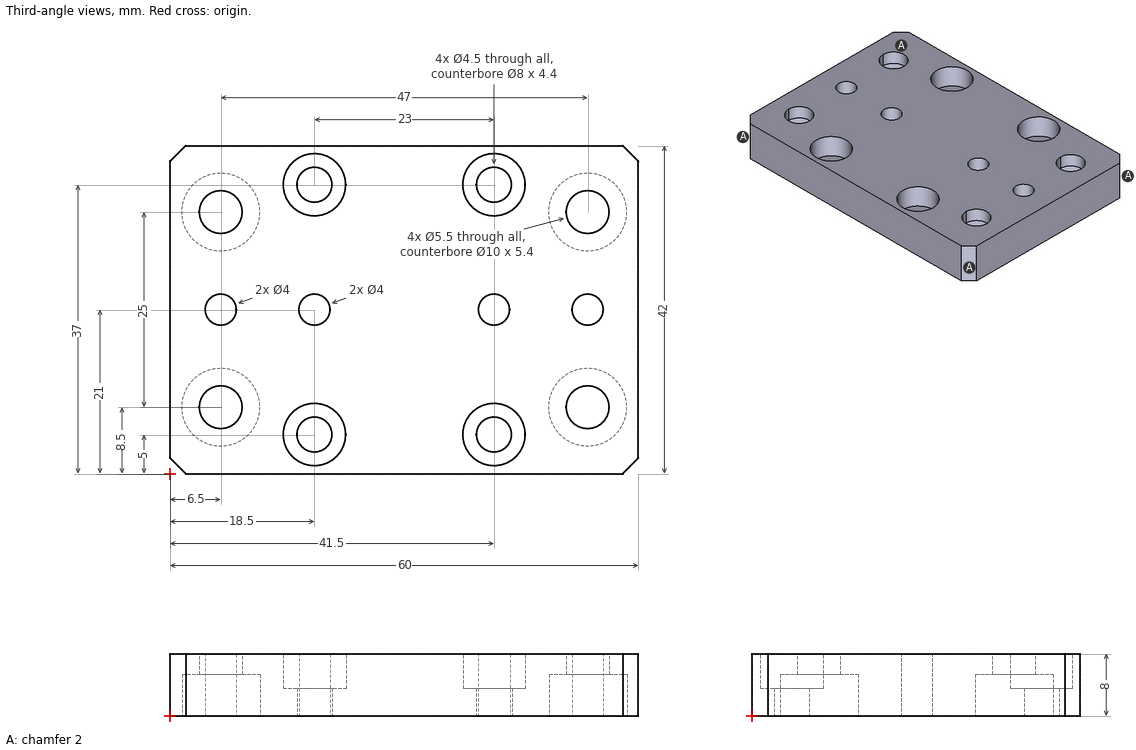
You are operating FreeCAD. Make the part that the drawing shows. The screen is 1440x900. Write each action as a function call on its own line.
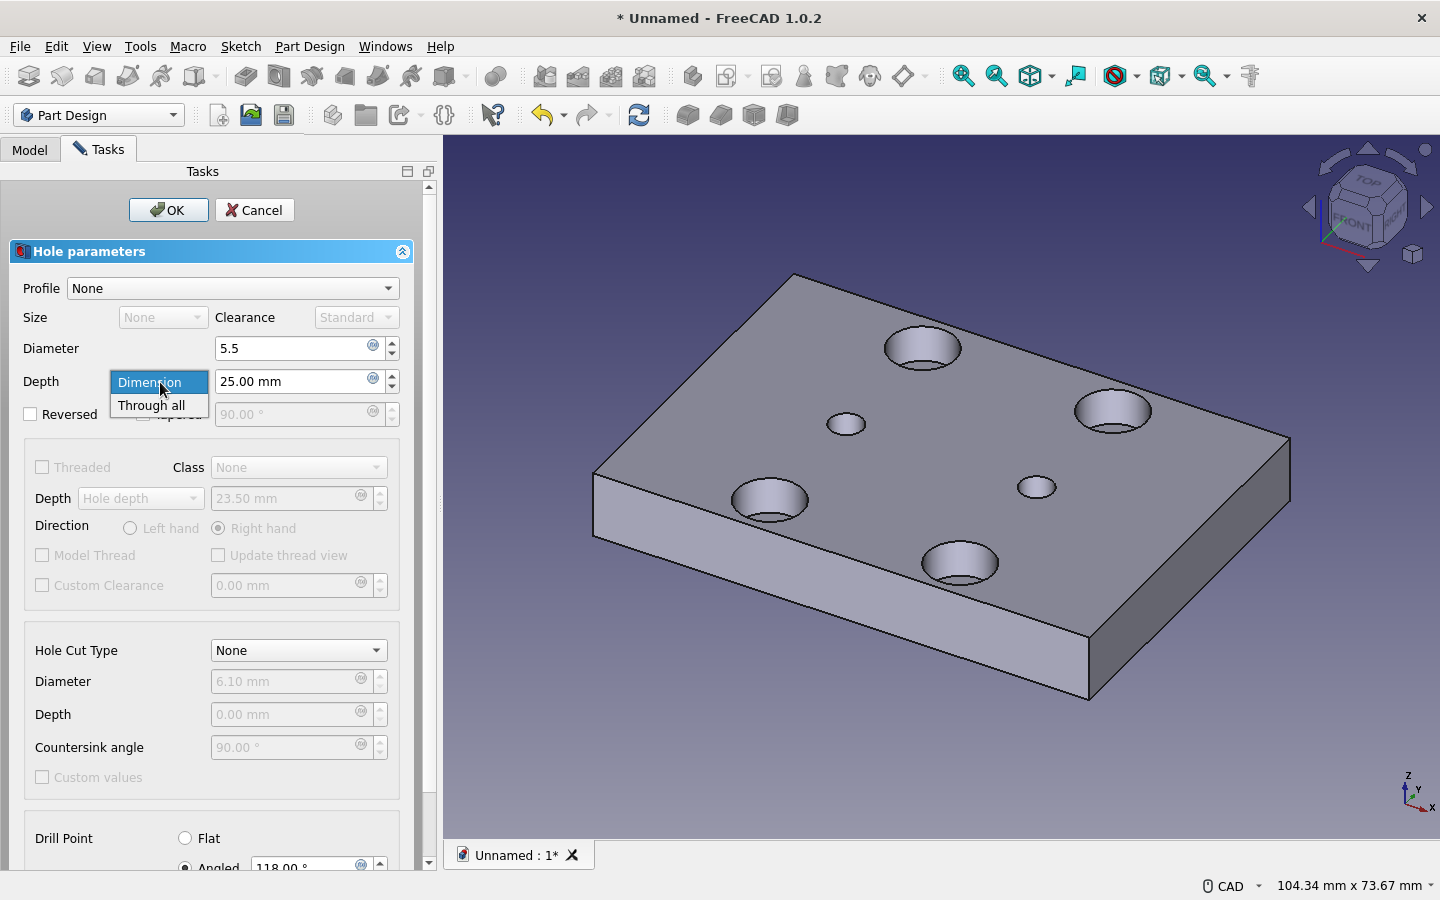
click(158, 406)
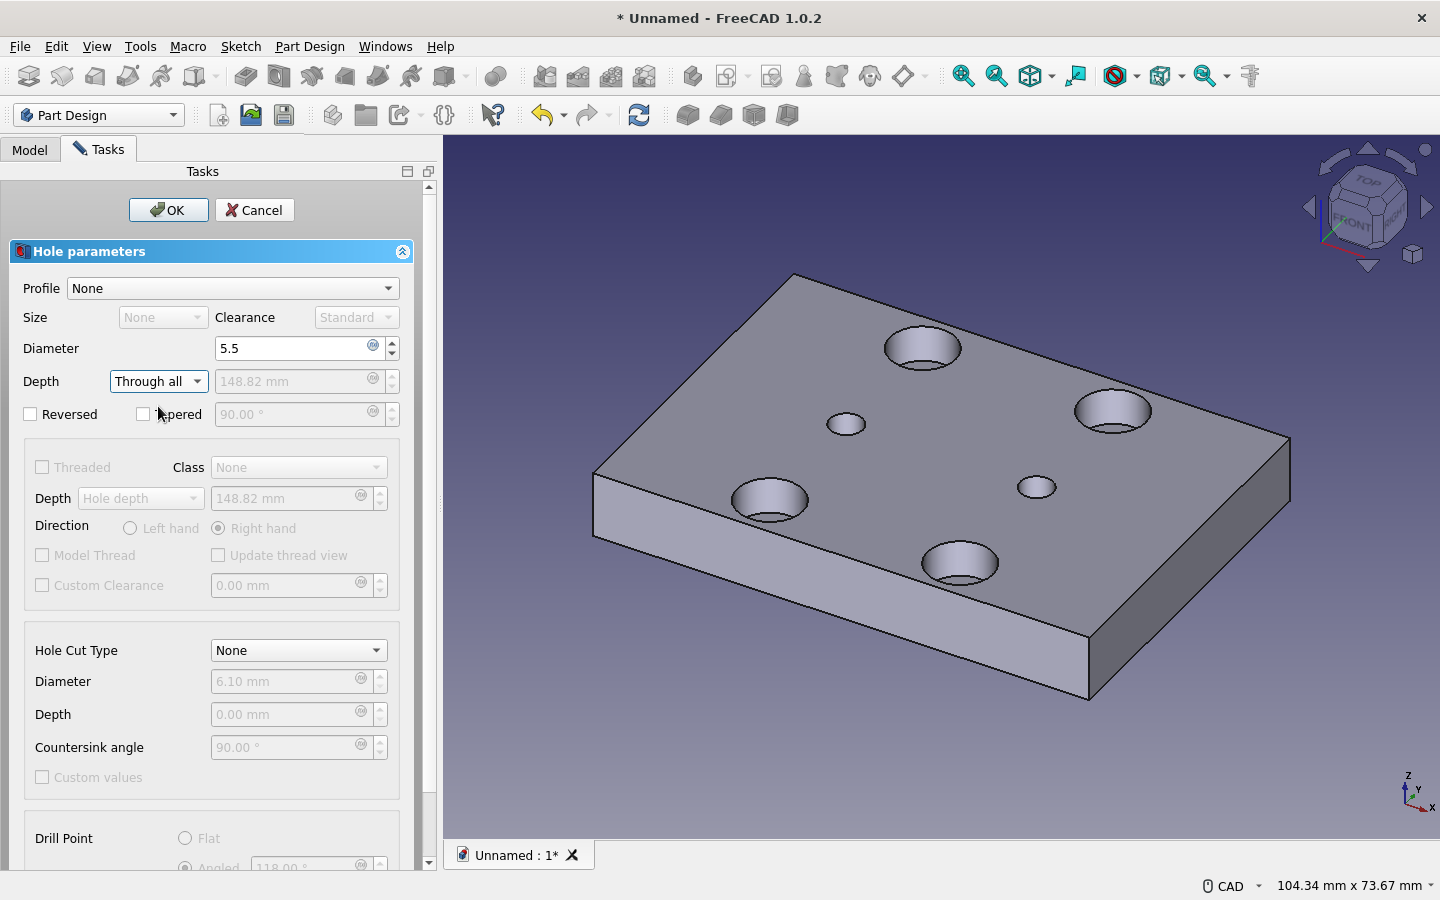
click(31, 414)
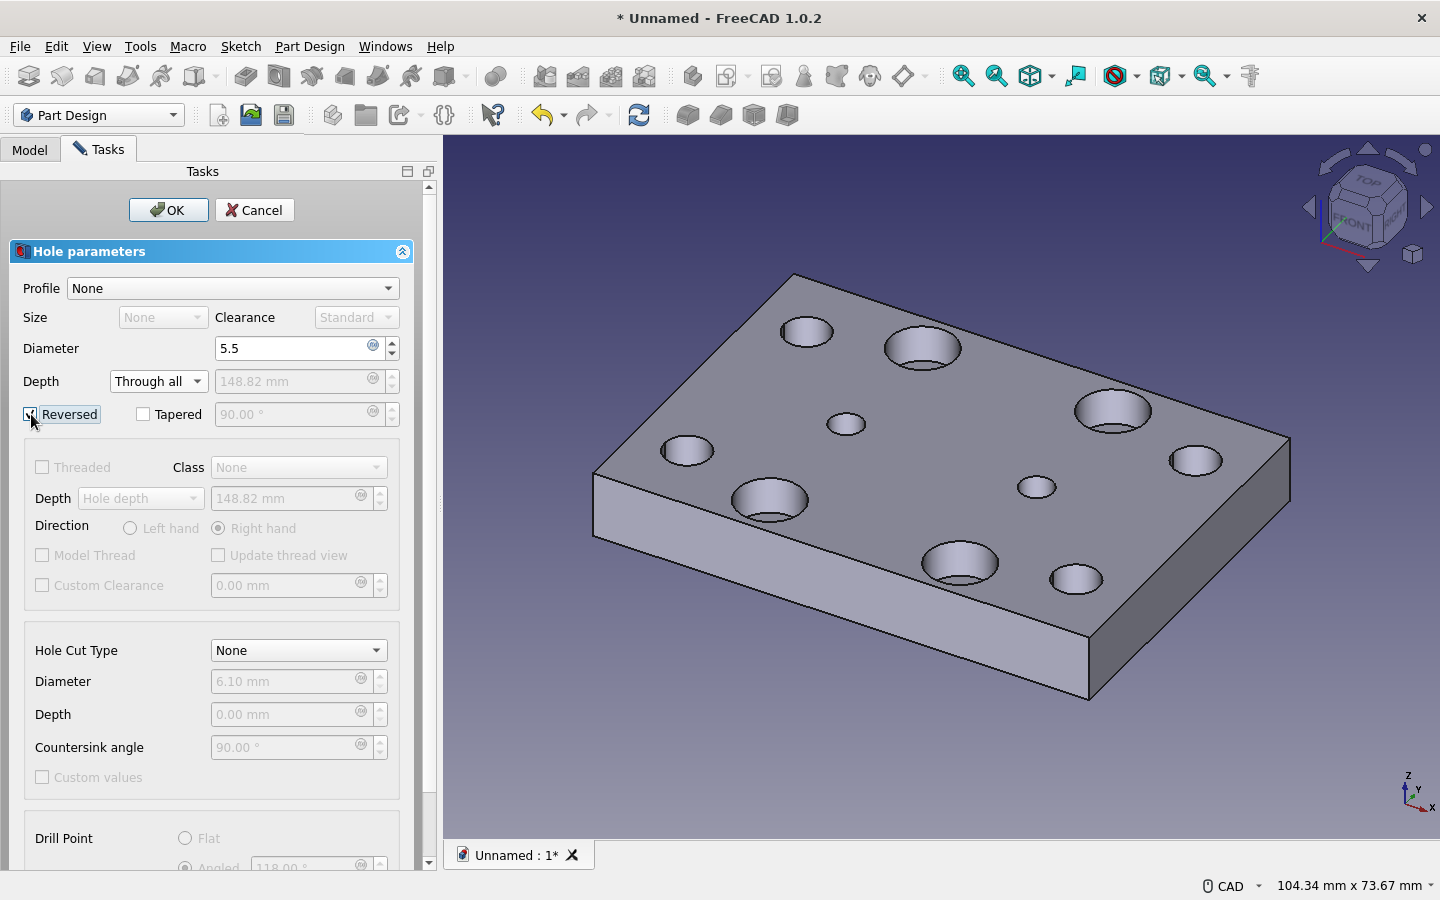
click(300, 650)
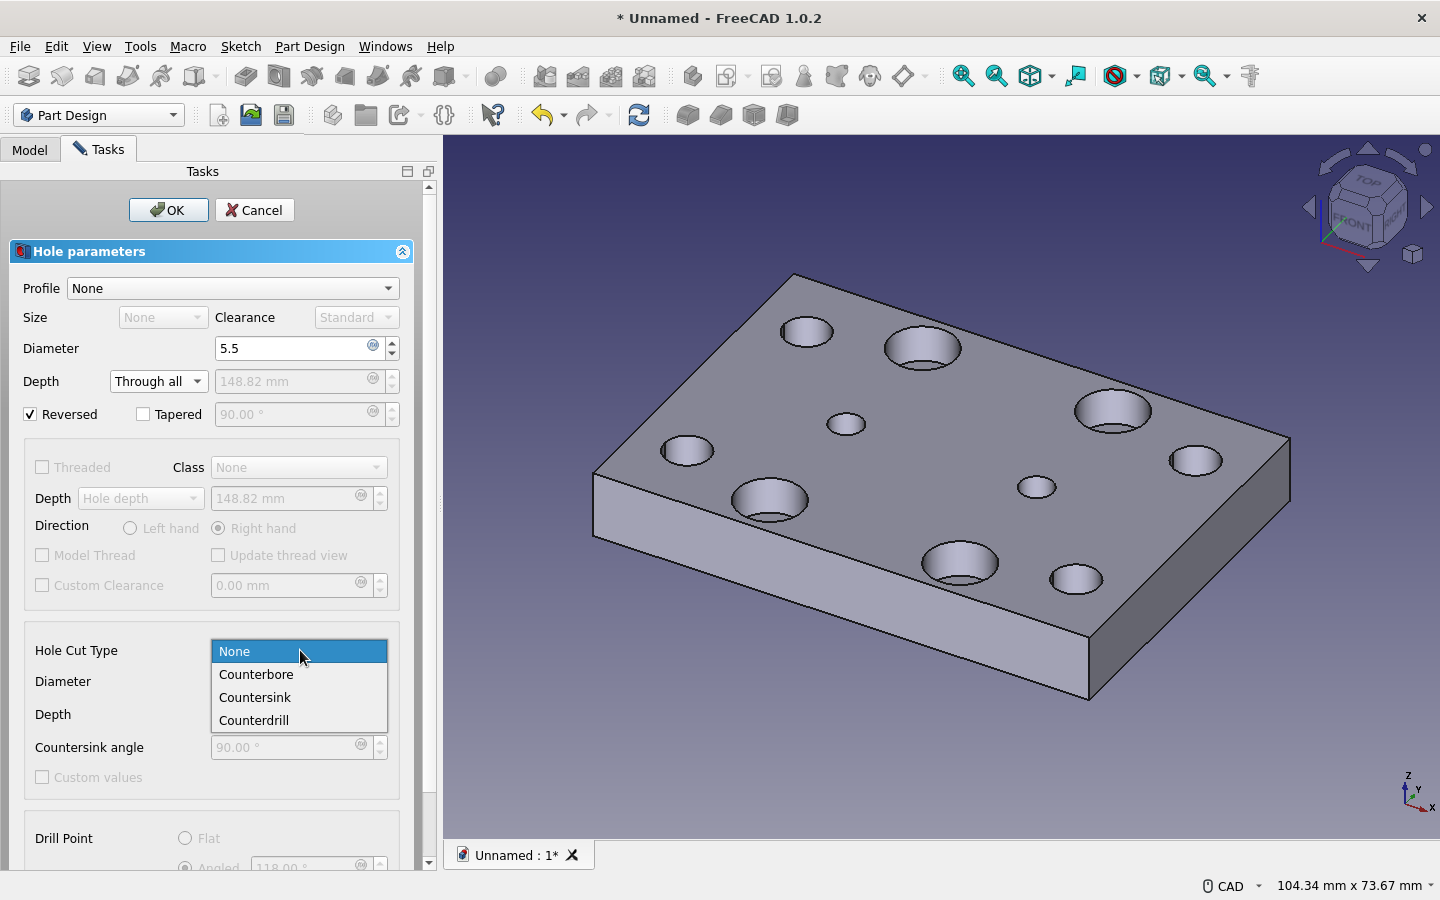
click(298, 674)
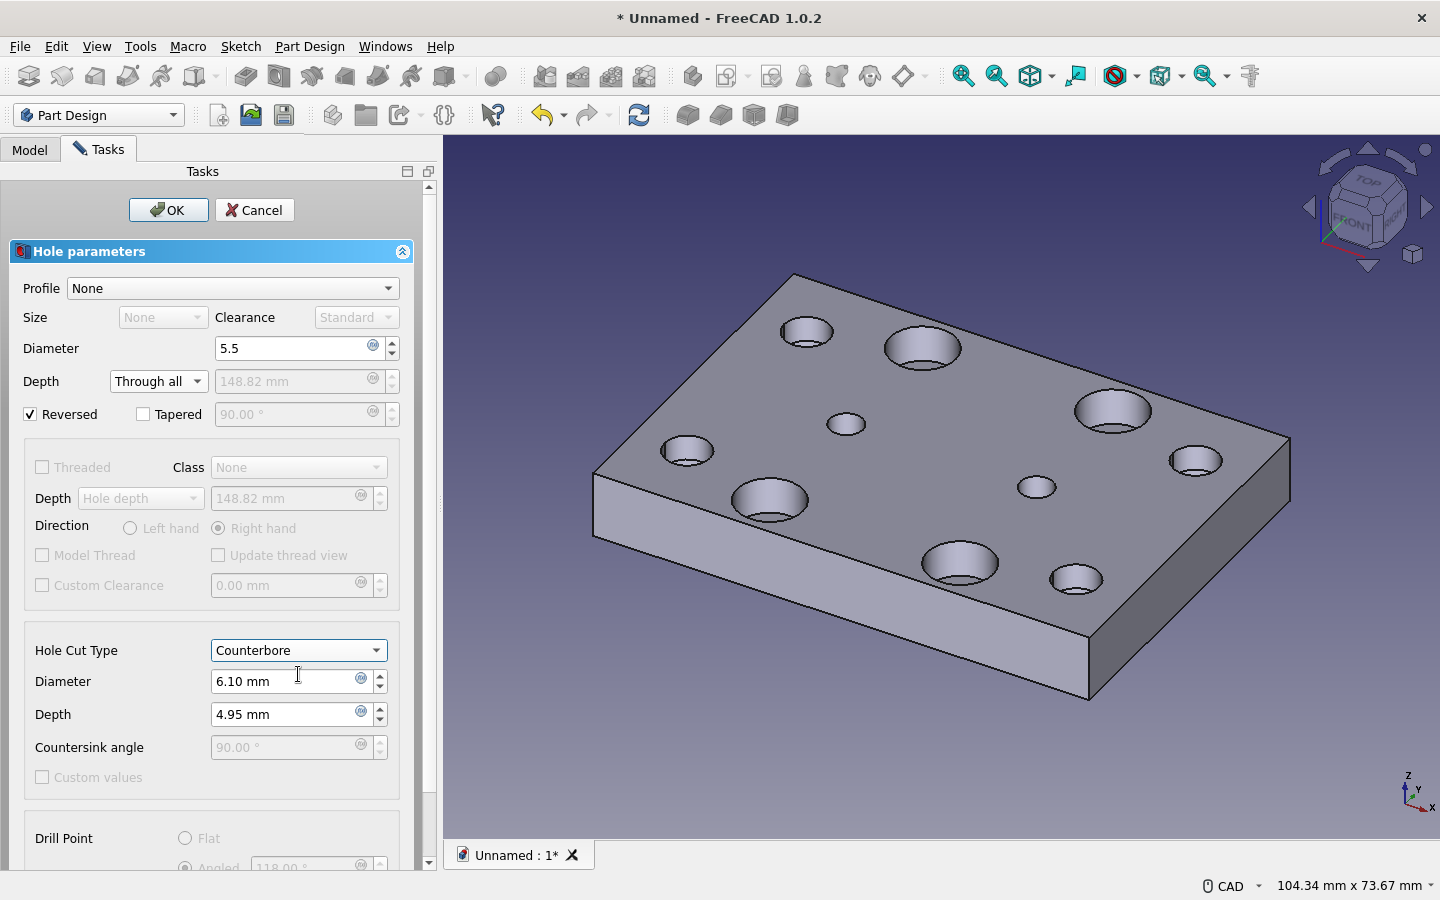
triple_click(292, 682)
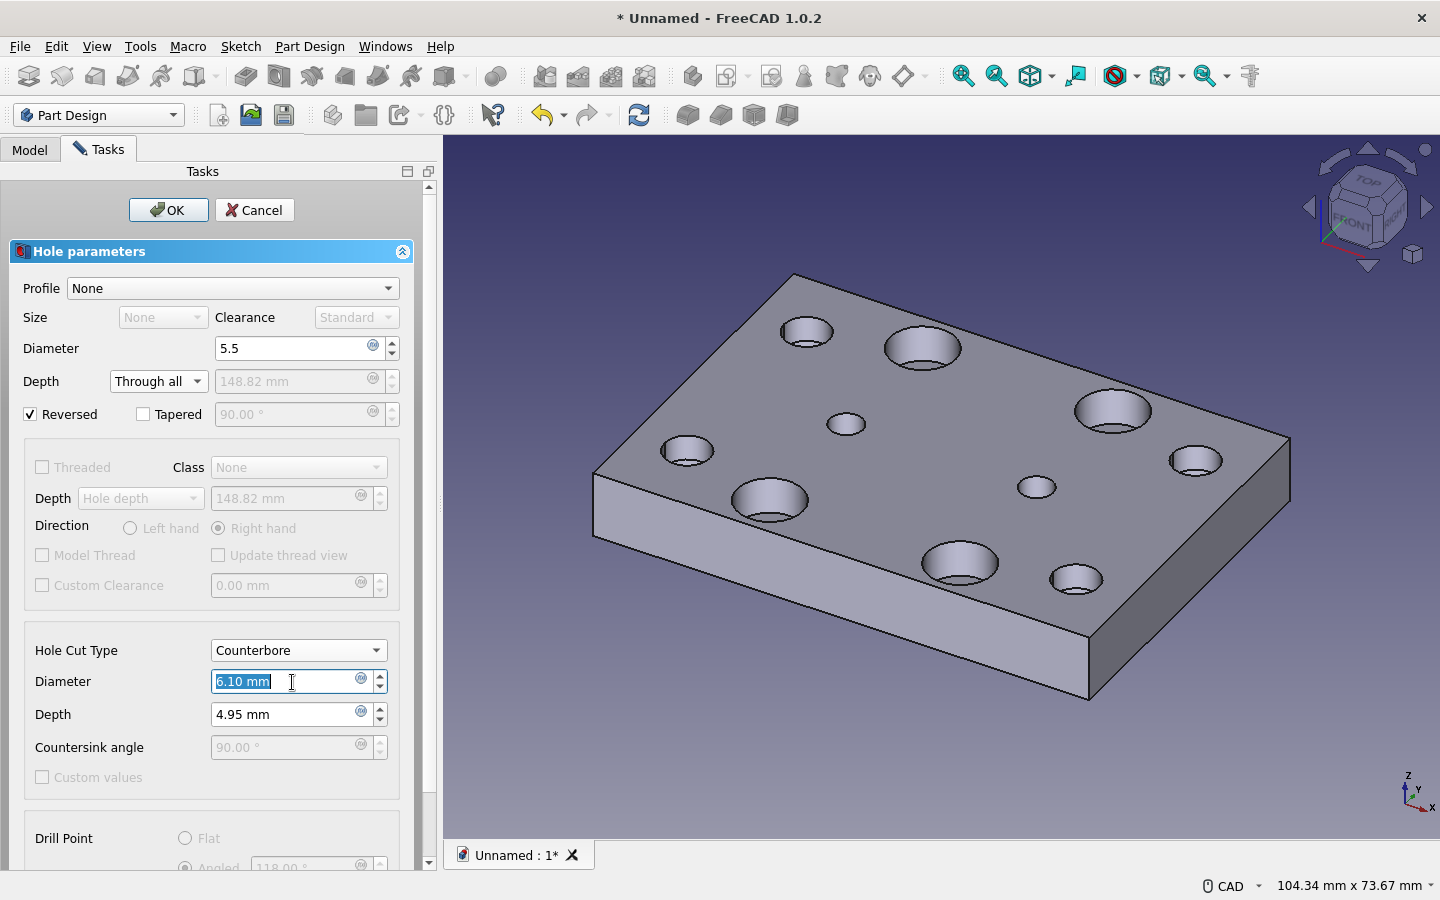
text(10)
key(Tab)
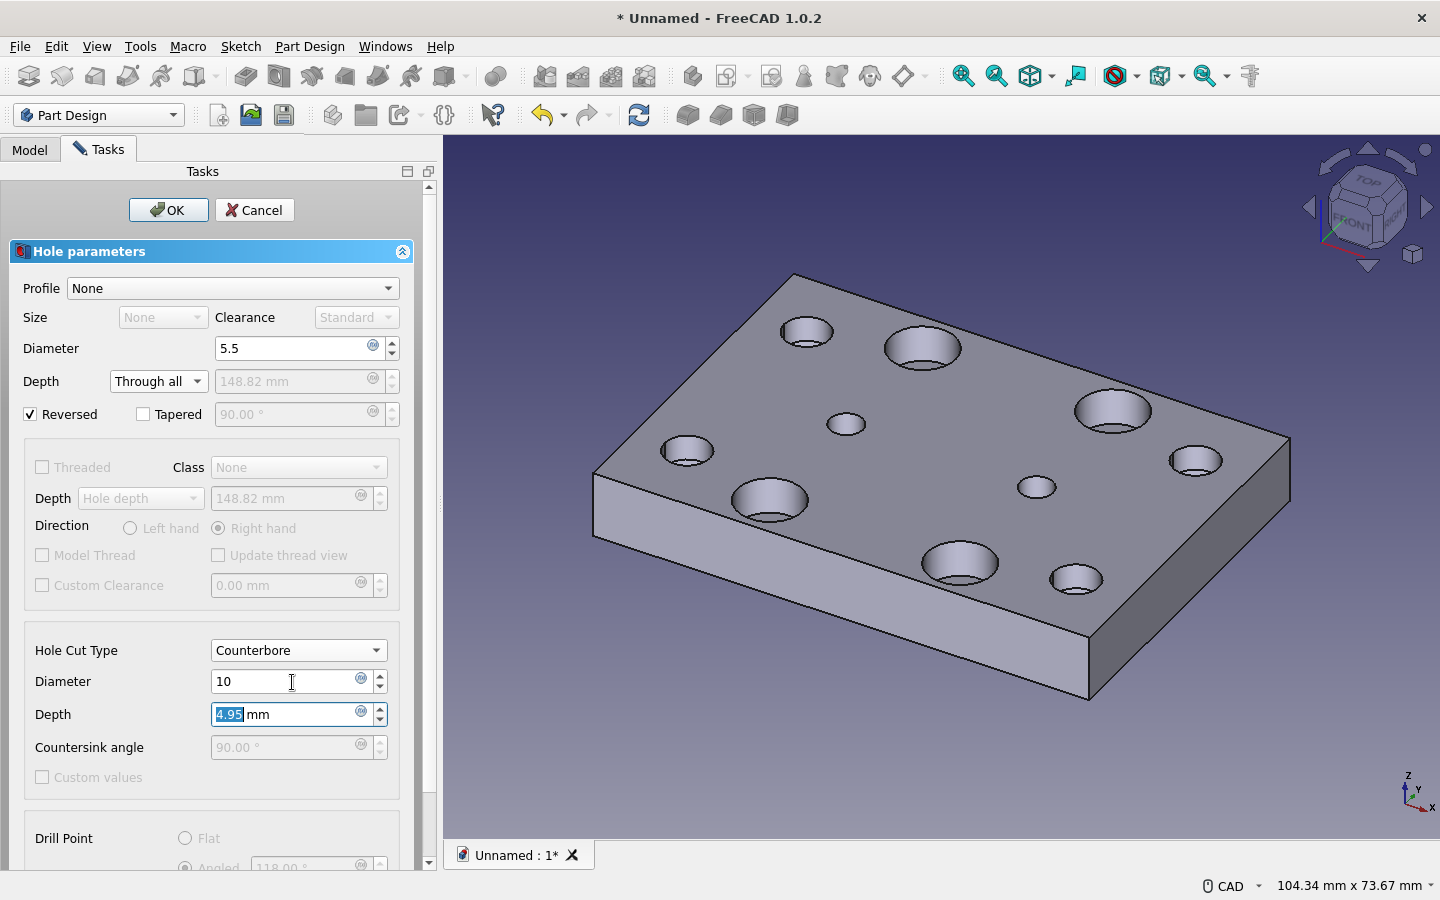
text(5.4)
key(Tab)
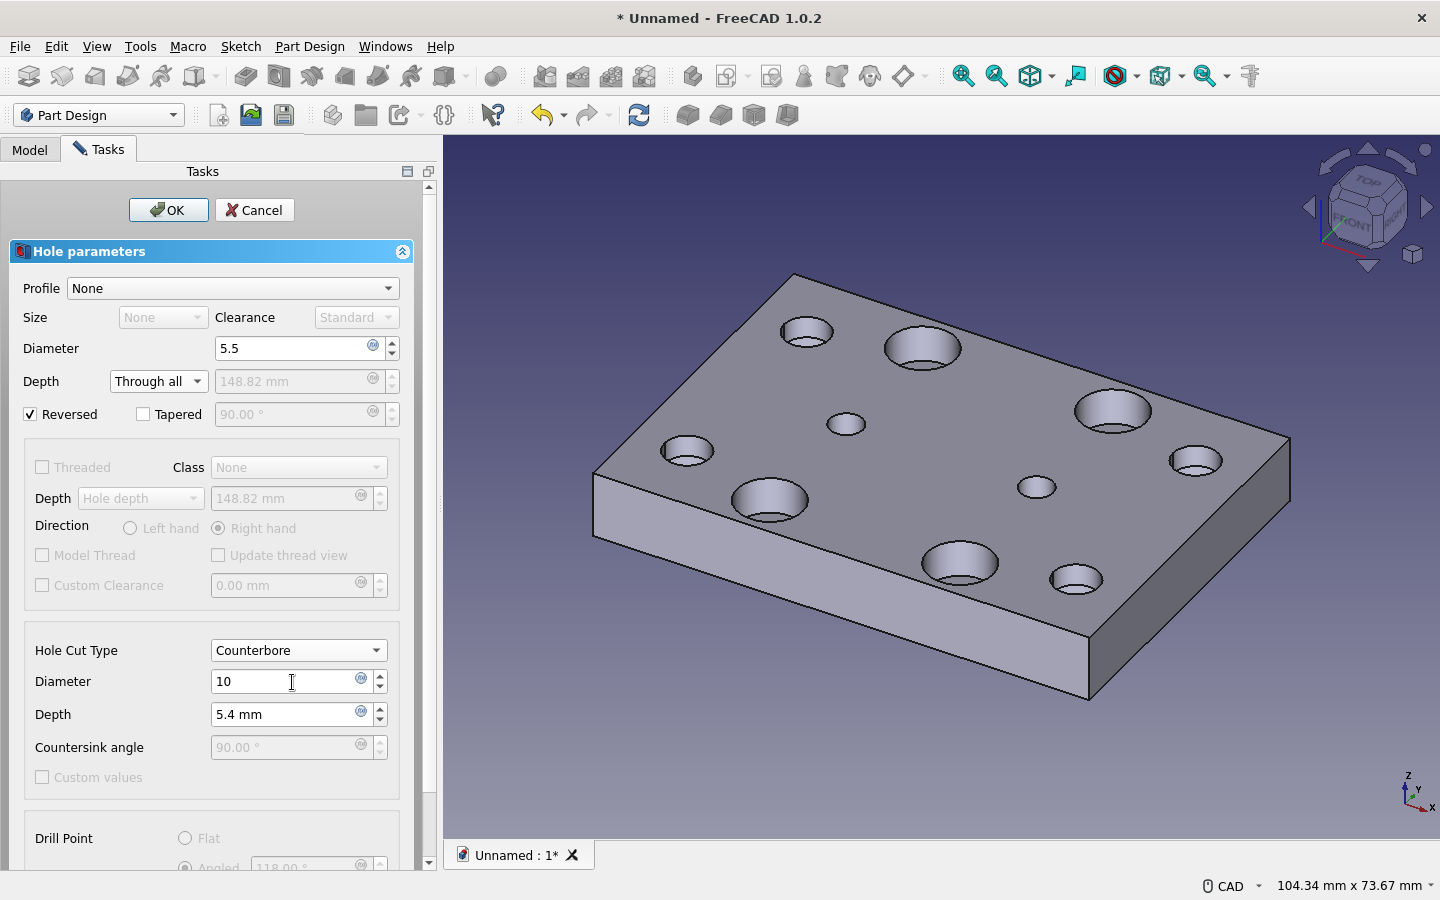
click(169, 210)